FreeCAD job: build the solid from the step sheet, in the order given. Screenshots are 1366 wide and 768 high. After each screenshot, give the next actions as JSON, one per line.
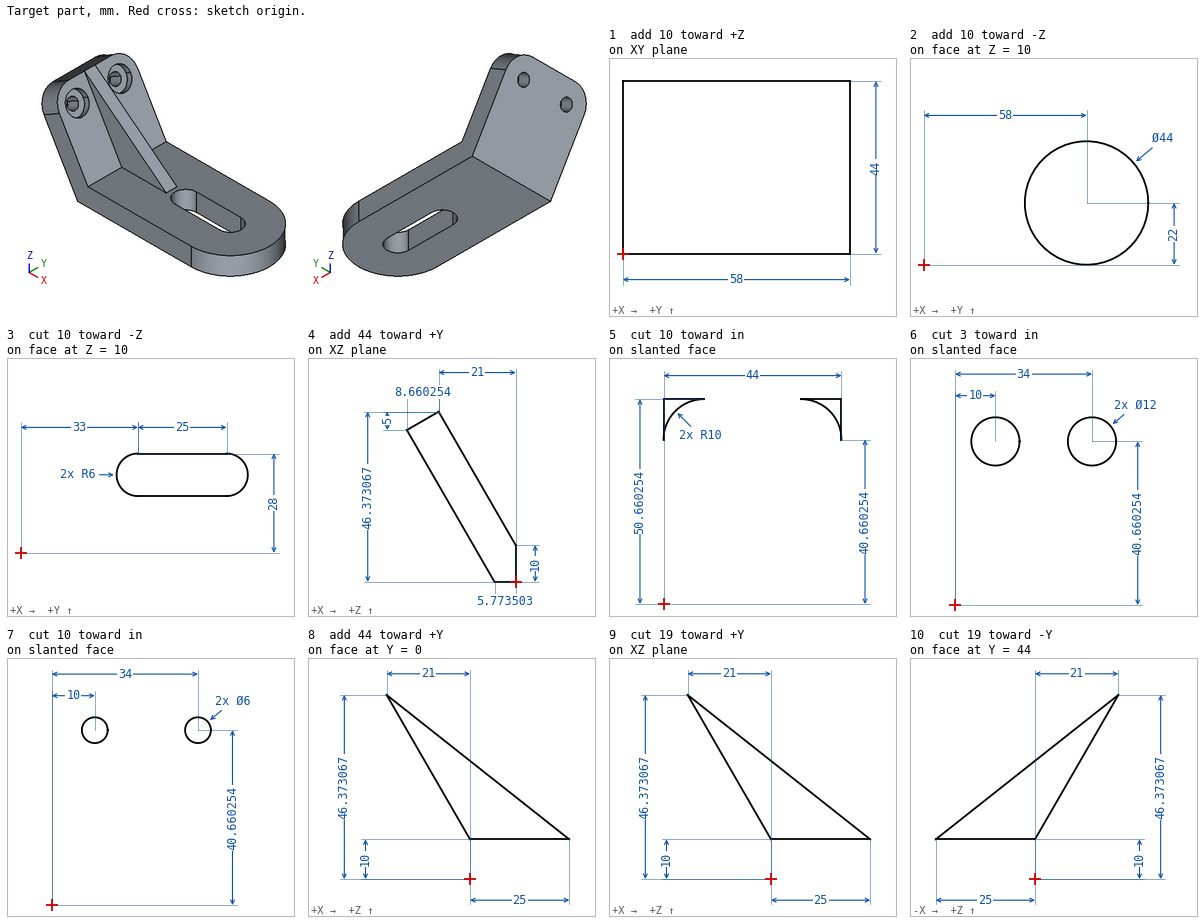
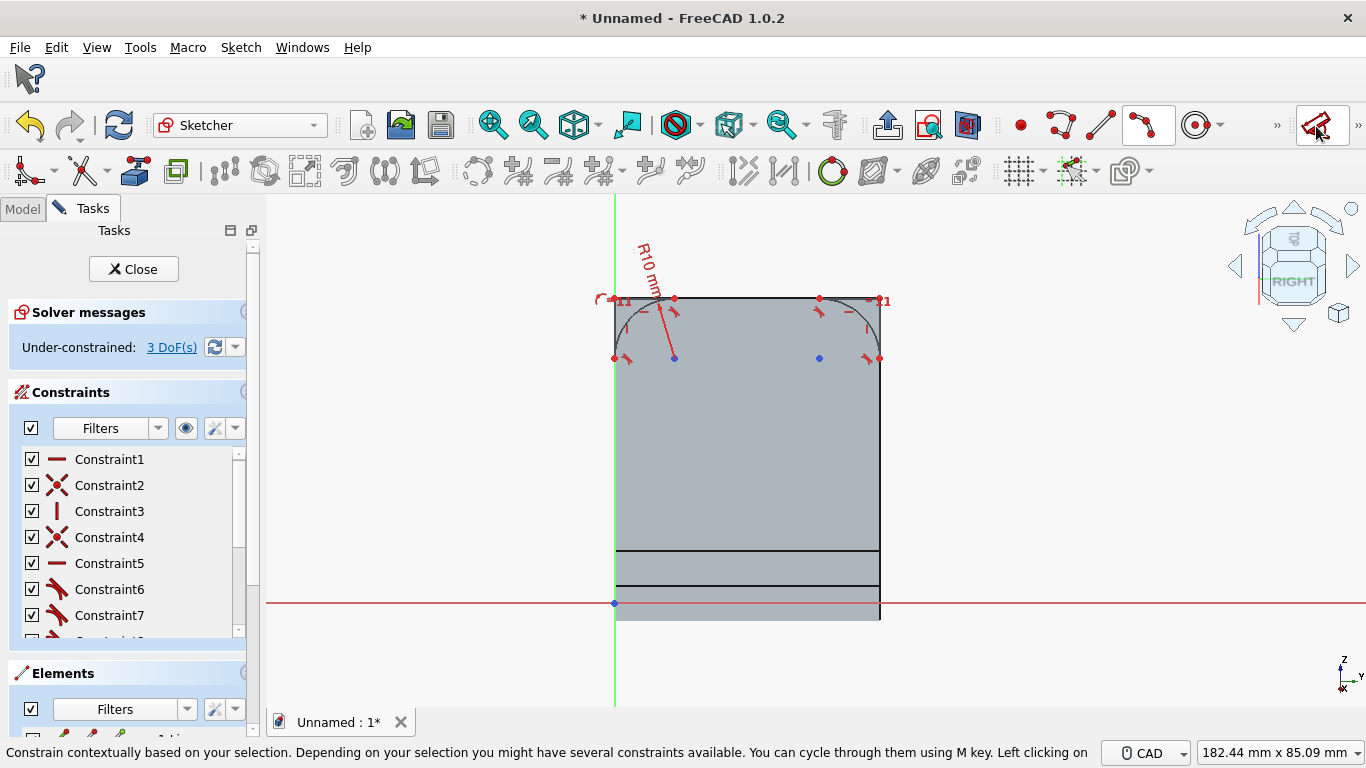
{"action": "left_click", "coordinate": [880, 359]}
{"action": "left_click", "coordinate": [747, 637]}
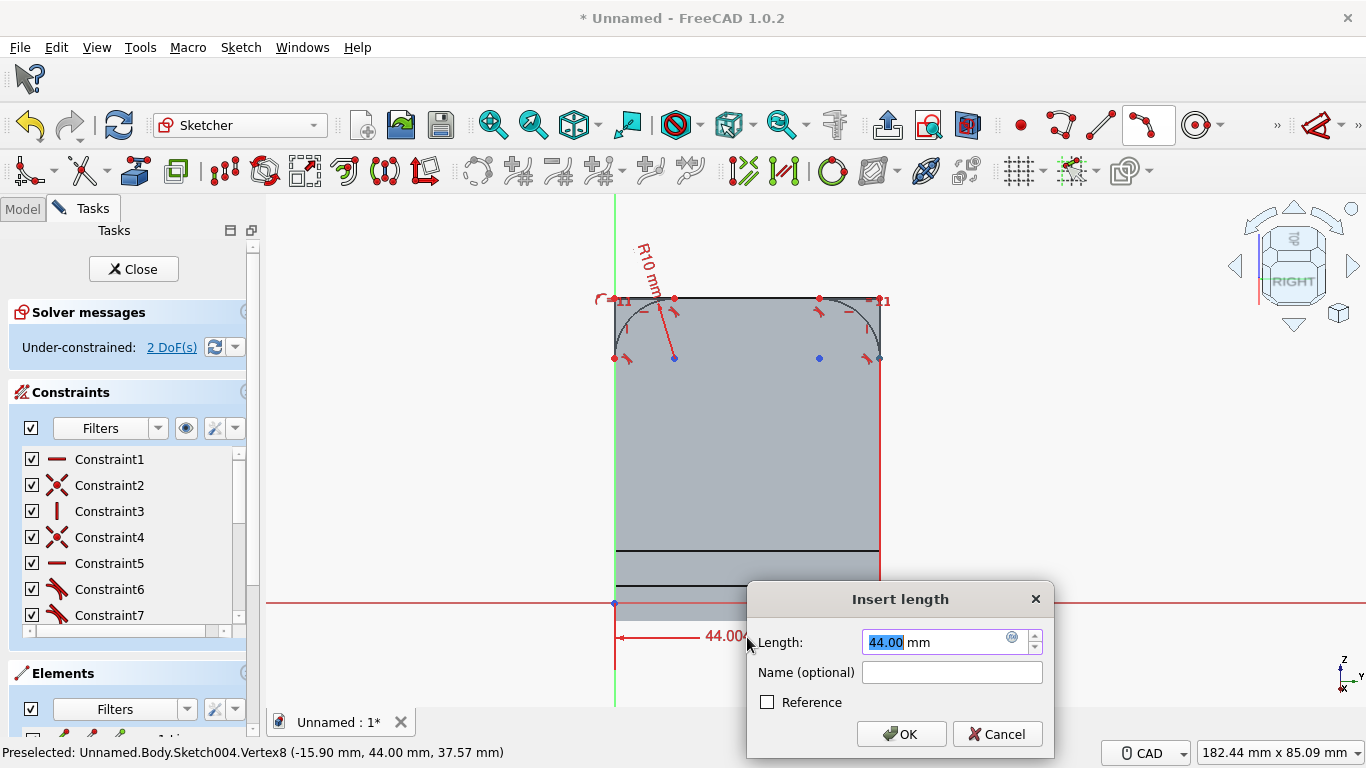
{"action": "type", "text": "44"}
{"action": "key", "text": "Return"}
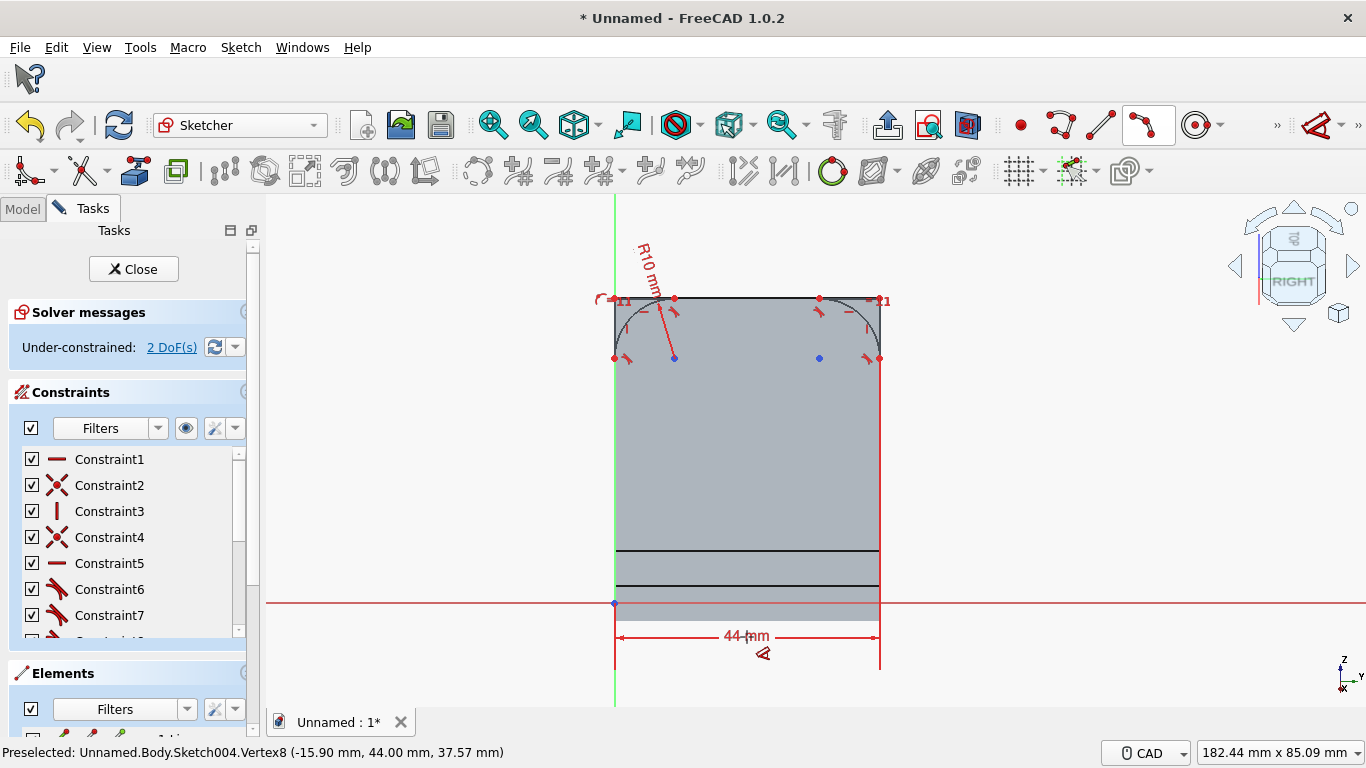
{"action": "left_click", "coordinate": [675, 299]}
{"action": "left_click", "coordinate": [581, 451]}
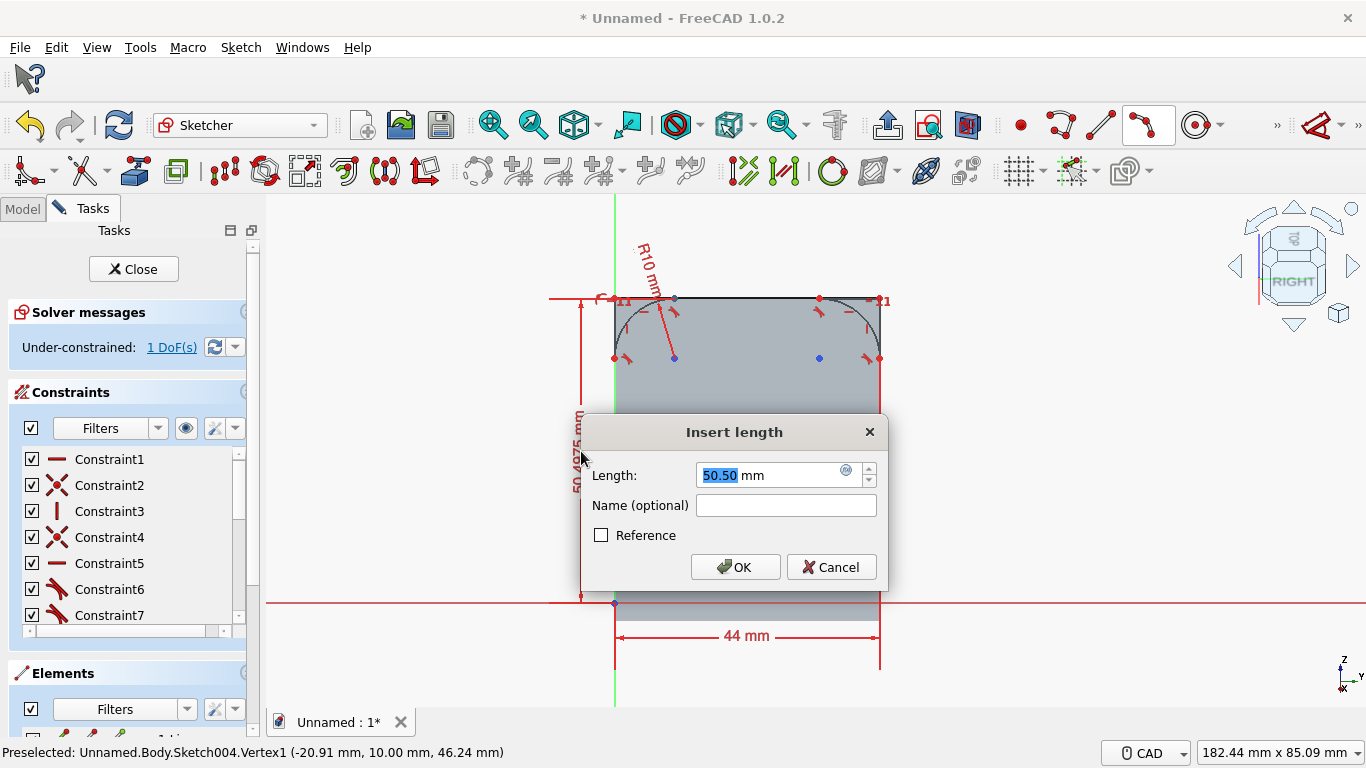
{"action": "type", "text": "50.660254"}
{"action": "key", "text": "Return"}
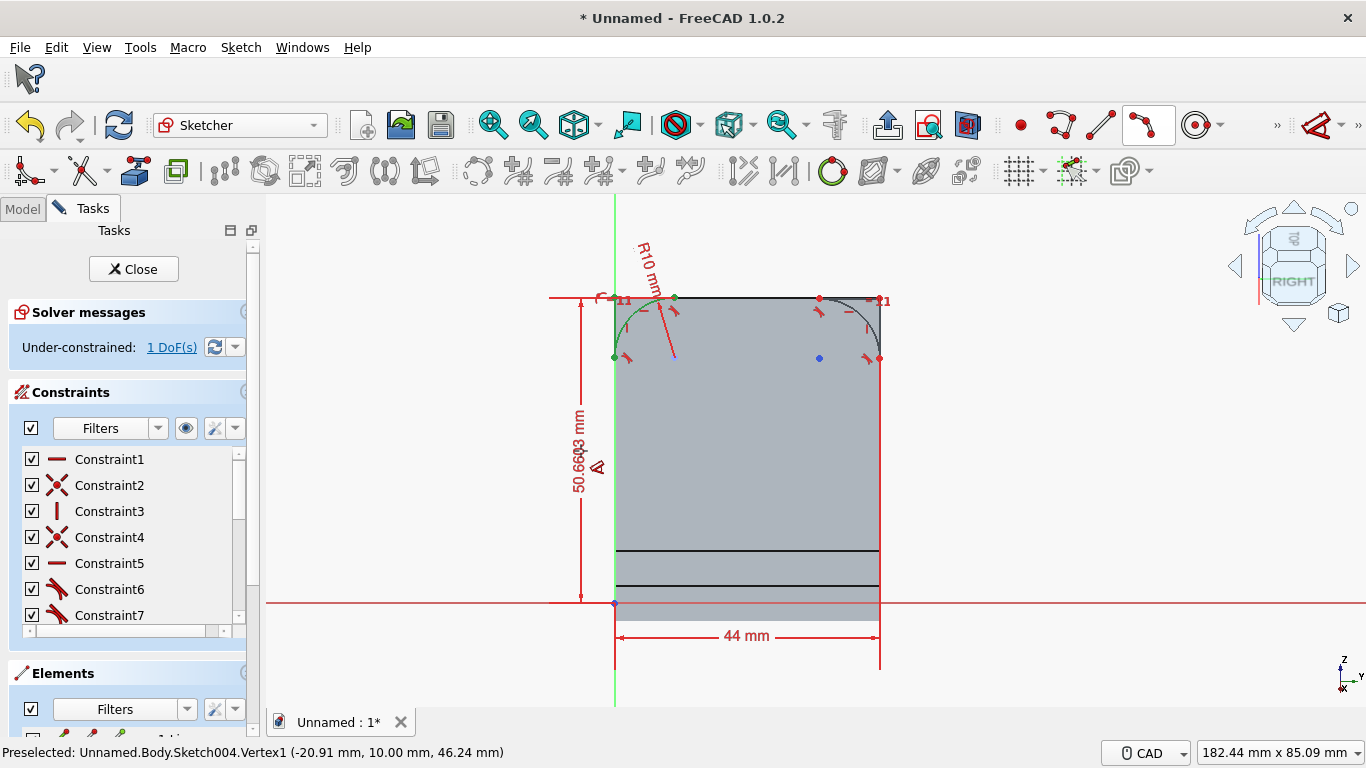
{"action": "left_click", "coordinate": [880, 359]}
{"action": "left_click", "coordinate": [581, 481]}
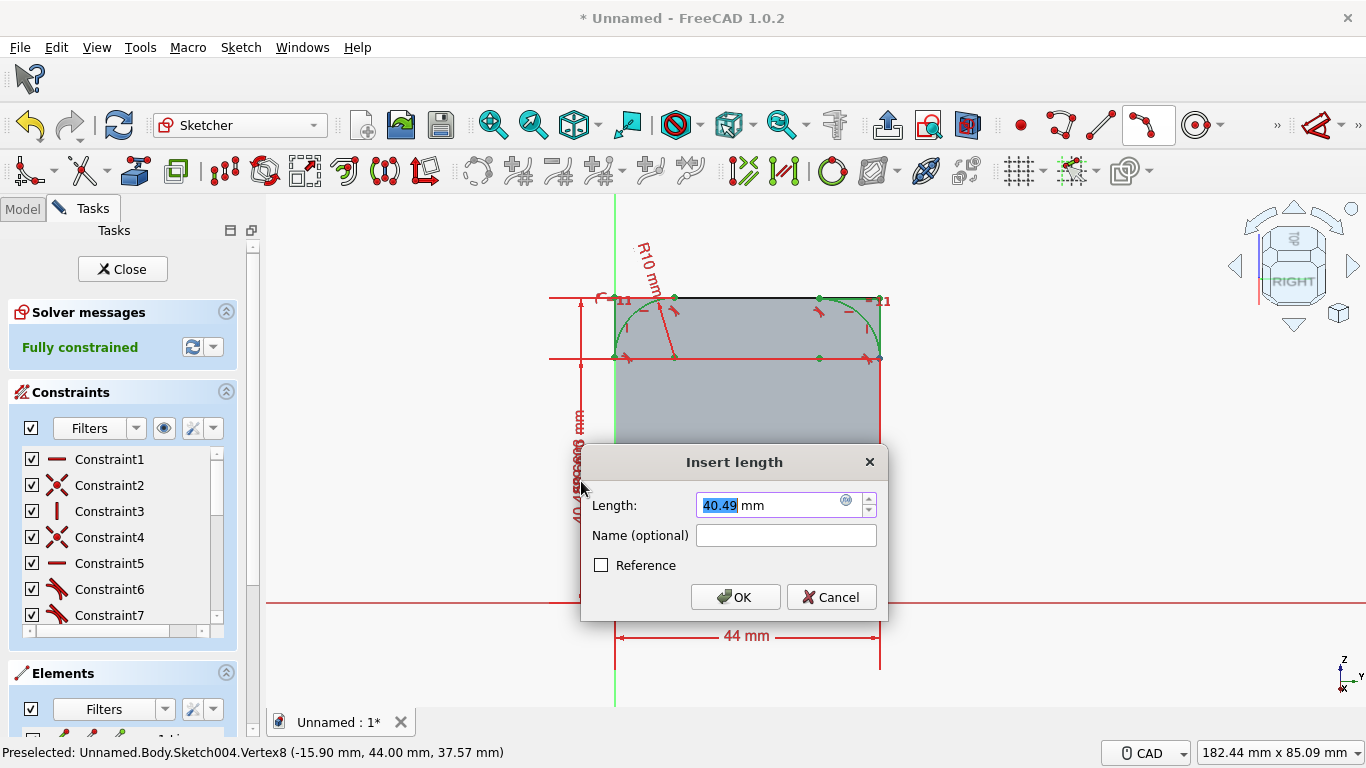
{"action": "type", "text": "40.660254"}
{"action": "key", "text": "Return"}
{"action": "key", "text": "Escape"}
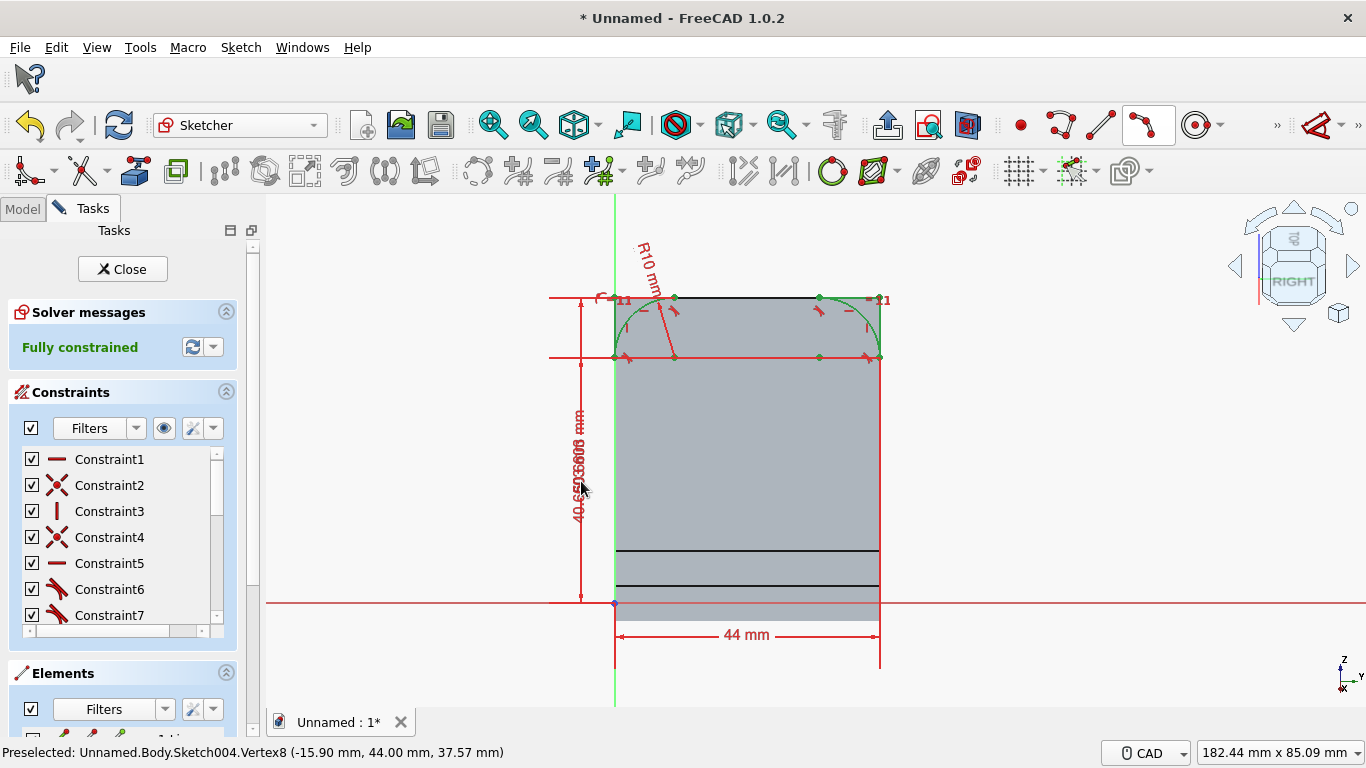
{"action": "left_click", "coordinate": [123, 269]}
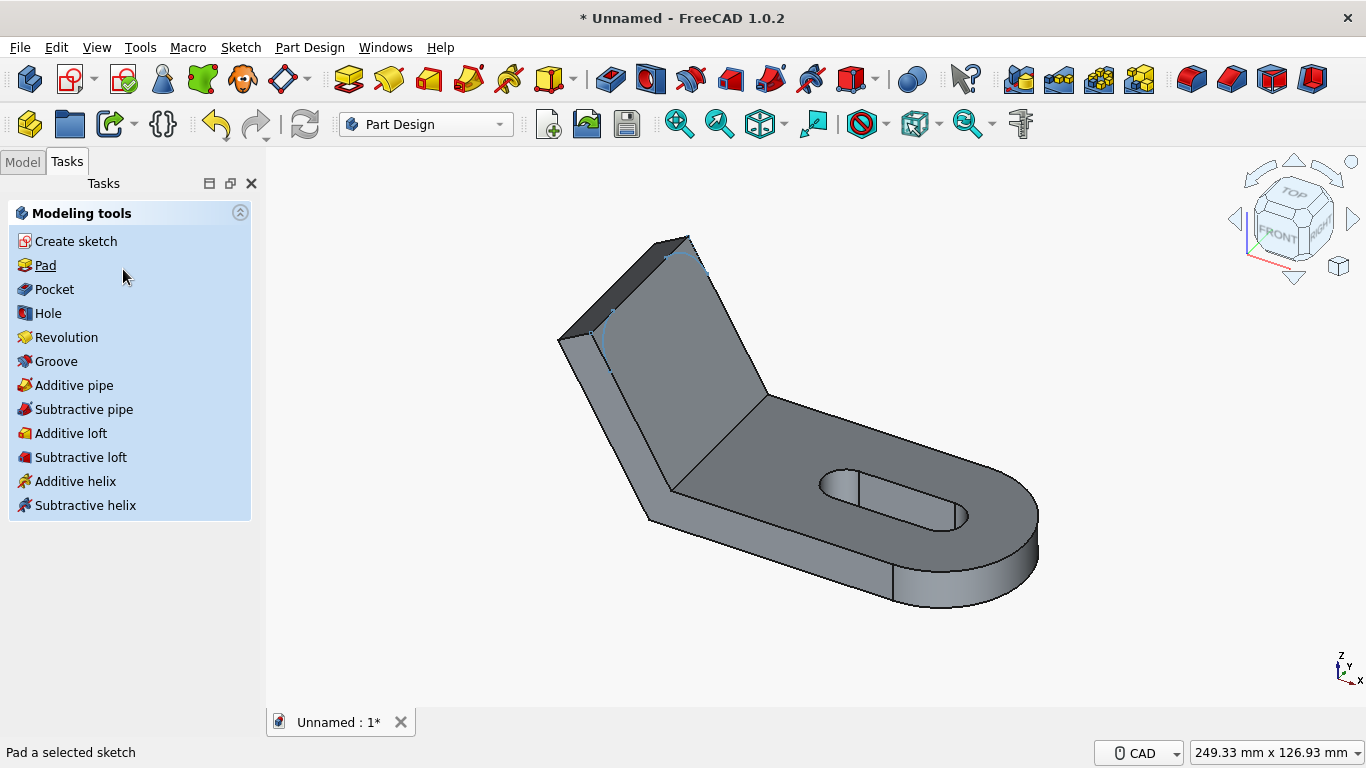
{"action": "left_click", "coordinate": [612, 80]}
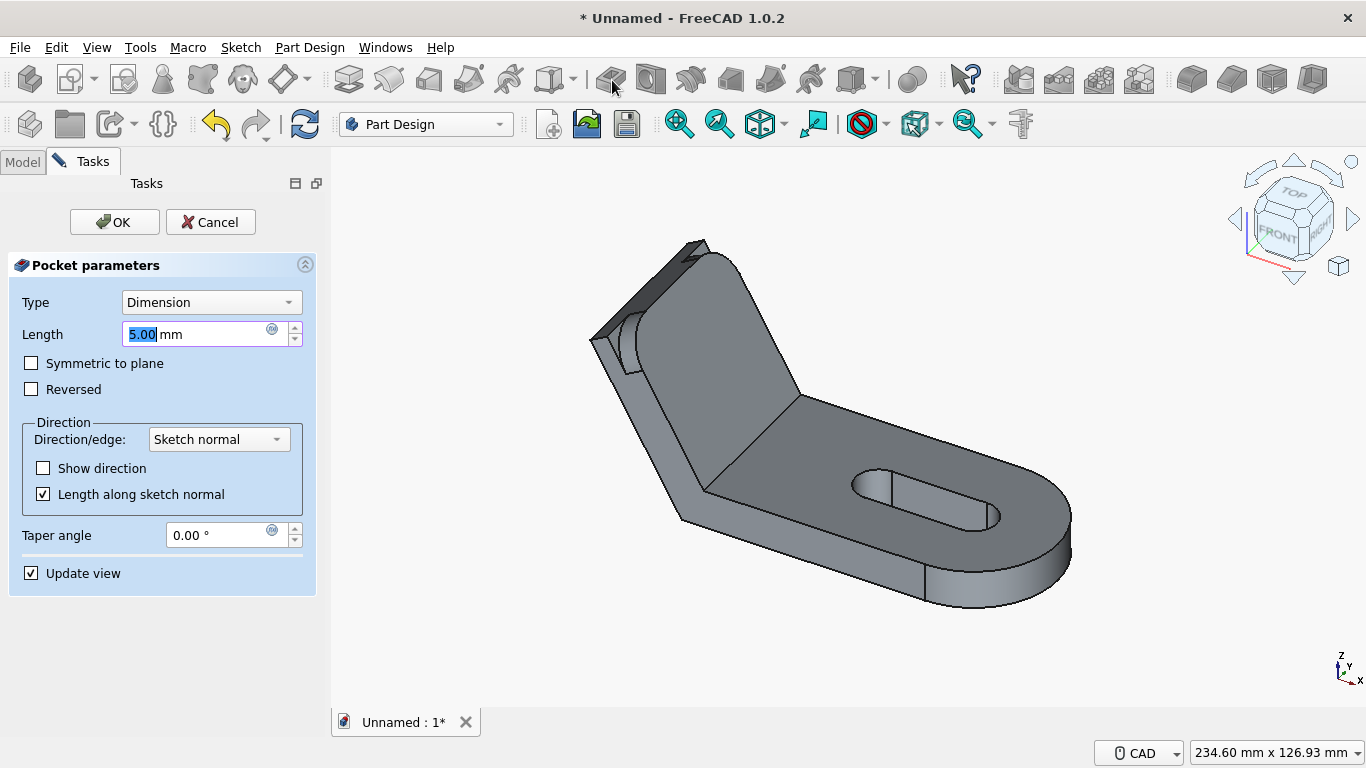
{"action": "type", "text": "10"}
{"action": "key", "text": "Tab"}